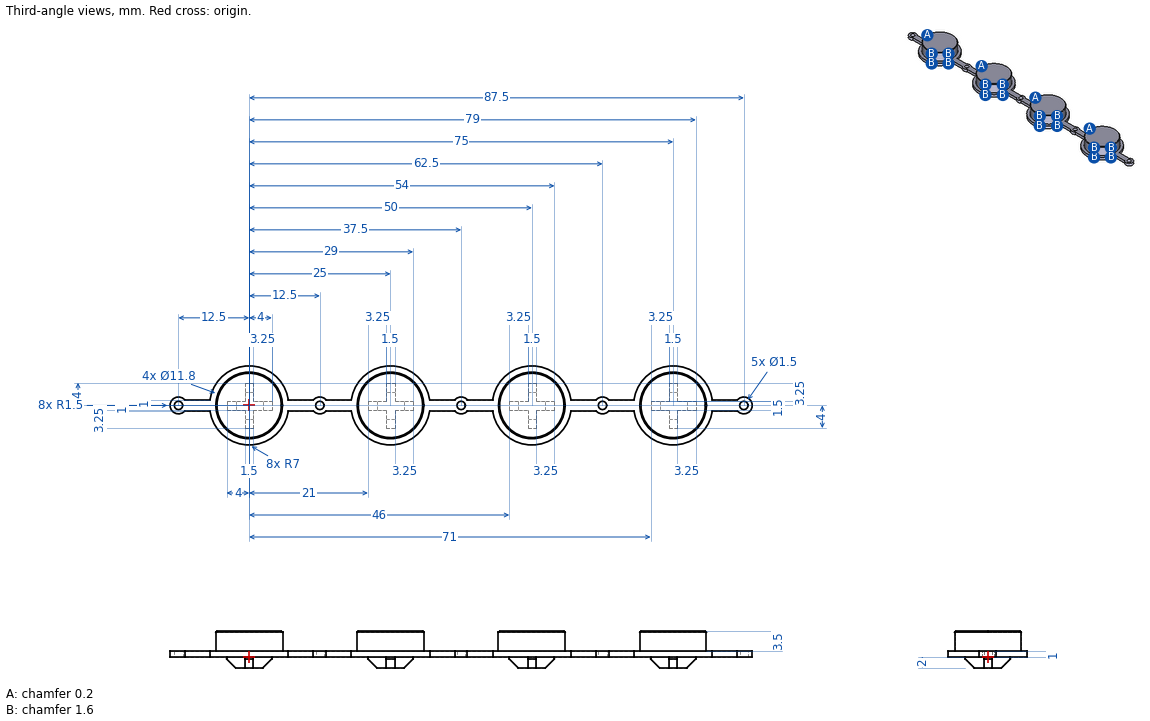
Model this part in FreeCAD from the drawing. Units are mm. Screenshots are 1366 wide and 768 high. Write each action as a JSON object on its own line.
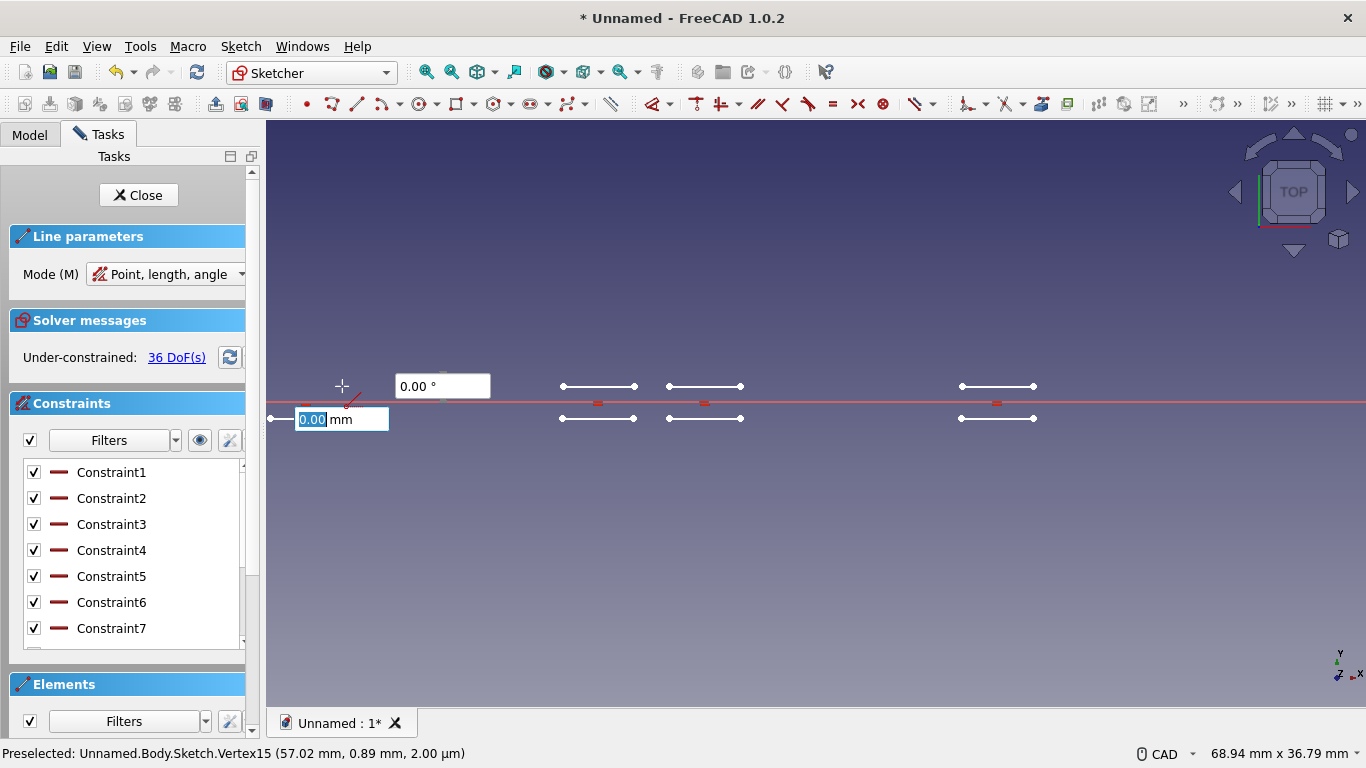
{"action": "scroll", "coordinate": [1036, 420], "scroll_direction": "down", "scroll_amount": 5}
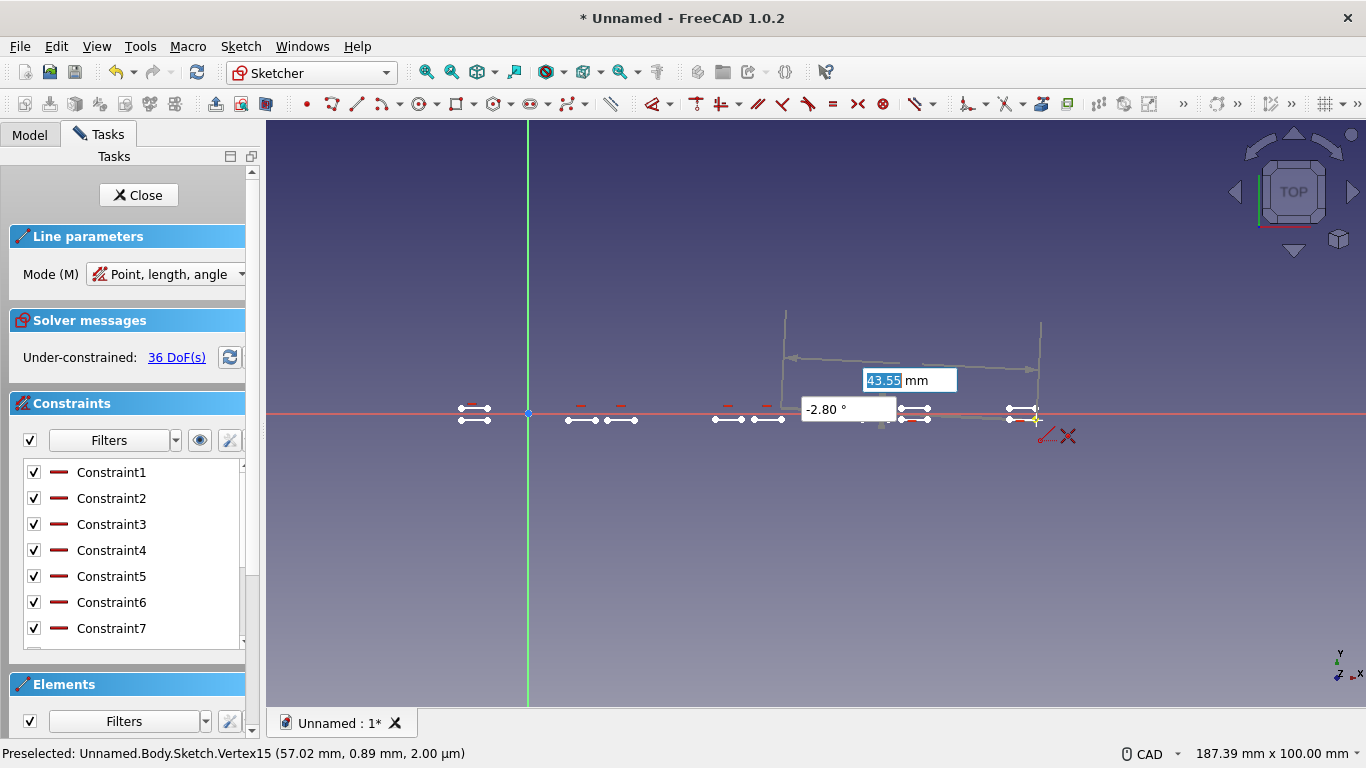
{"action": "scroll", "coordinate": [755, 408], "scroll_direction": "up", "scroll_amount": 5}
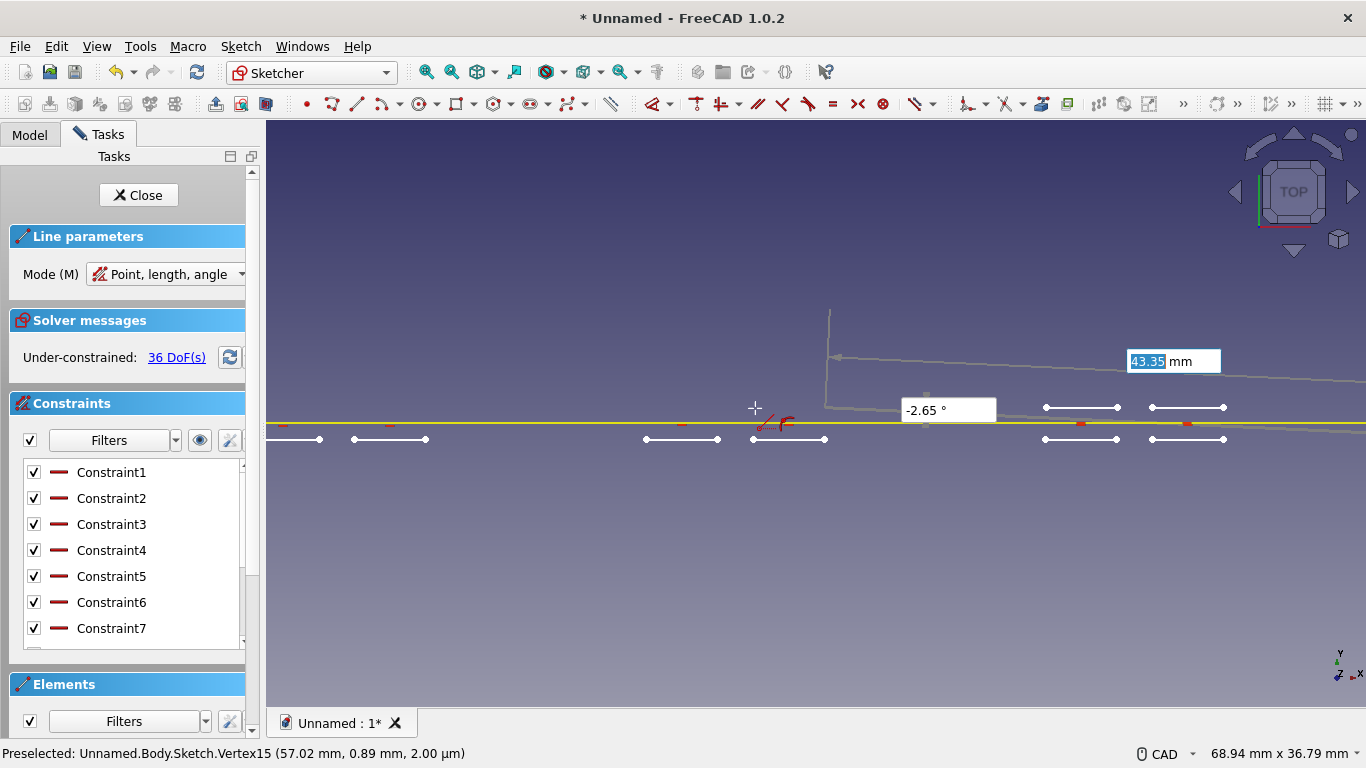
{"action": "left_click", "coordinate": [754, 407]}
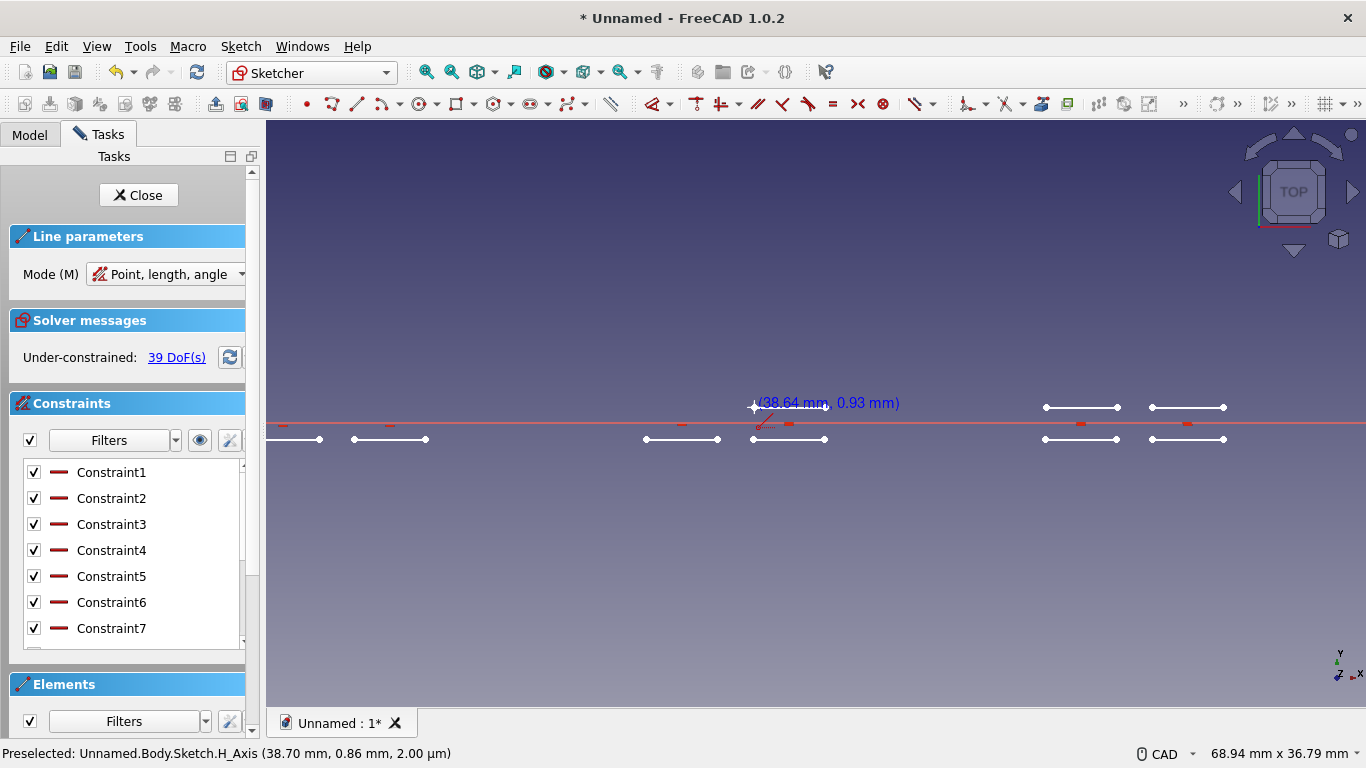
{"action": "left_click", "coordinate": [718, 407]}
{"action": "left_click", "coordinate": [647, 407]}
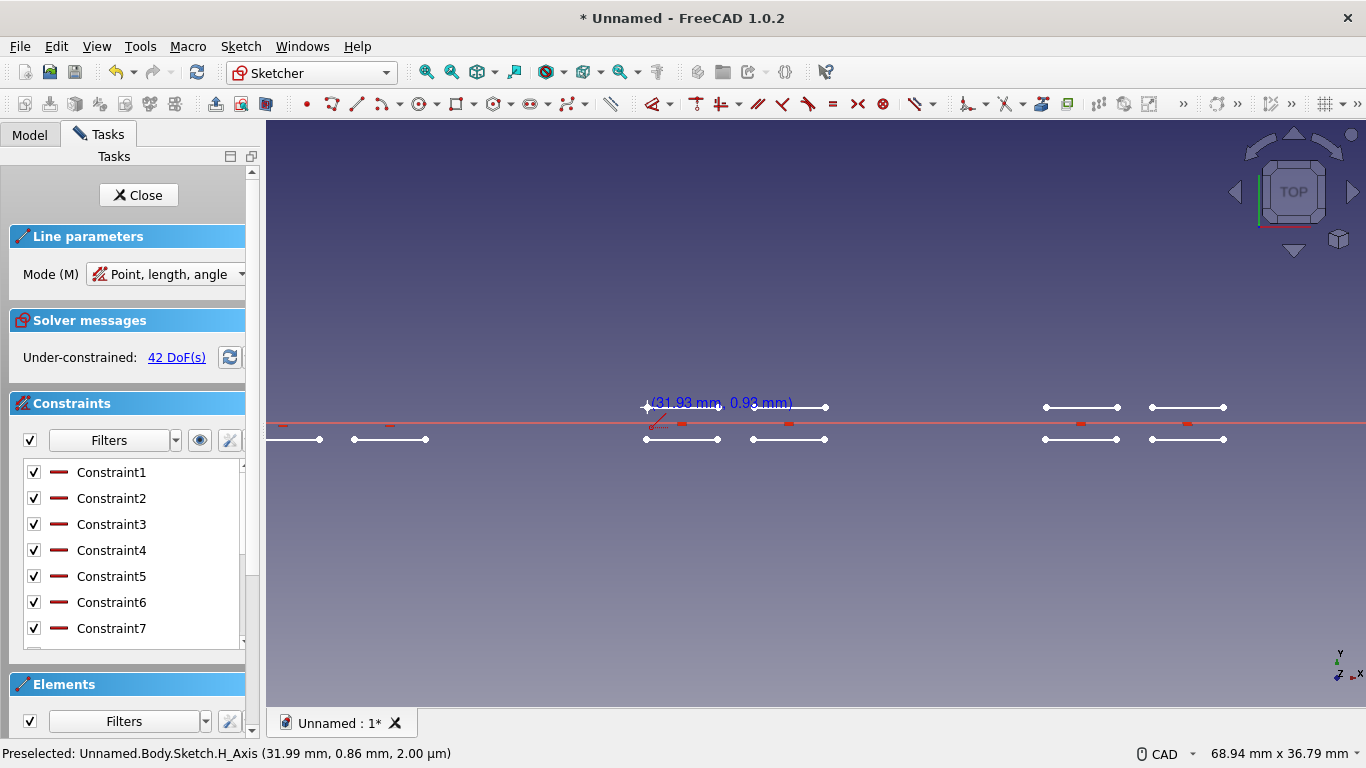
{"action": "left_click", "coordinate": [426, 407]}
{"action": "left_click", "coordinate": [355, 407]}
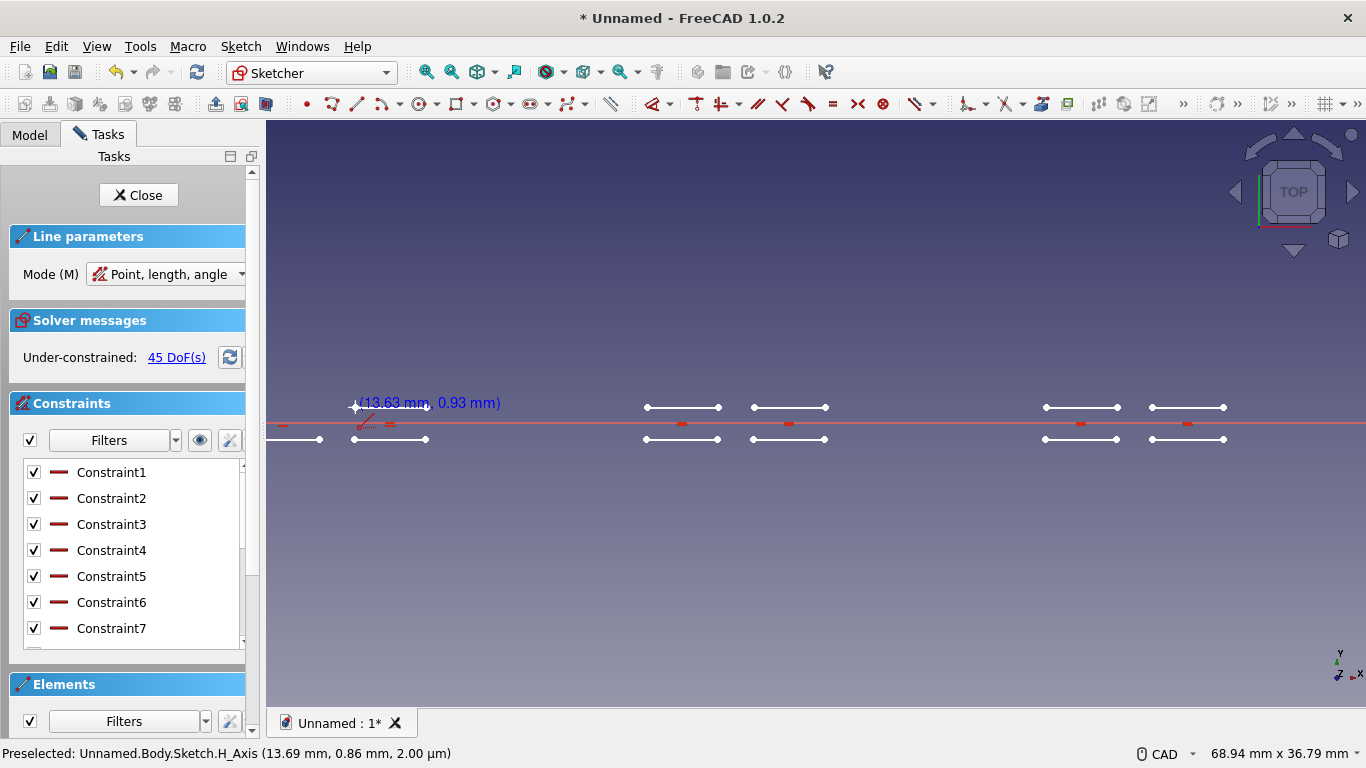
{"action": "left_click", "coordinate": [319, 407]}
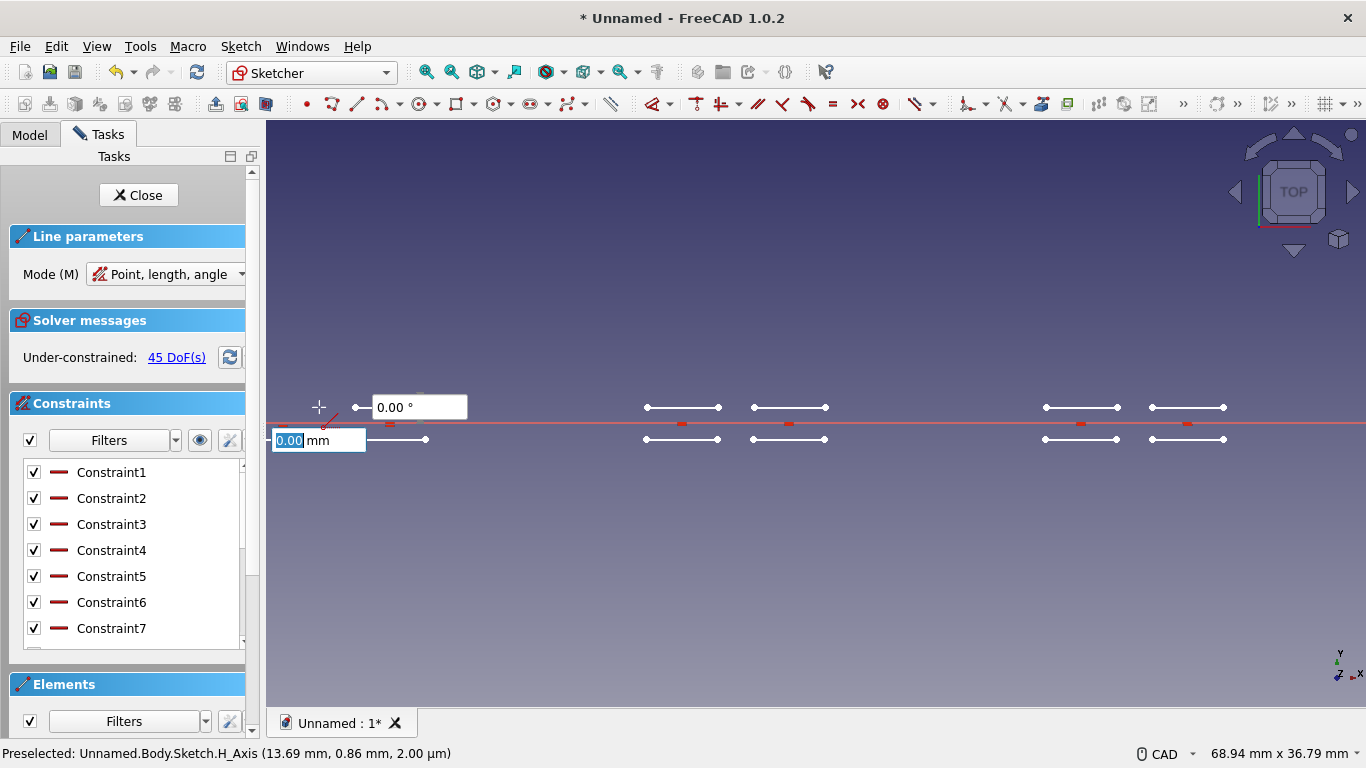
{"action": "scroll", "coordinate": [754, 408], "scroll_direction": "down", "scroll_amount": 5}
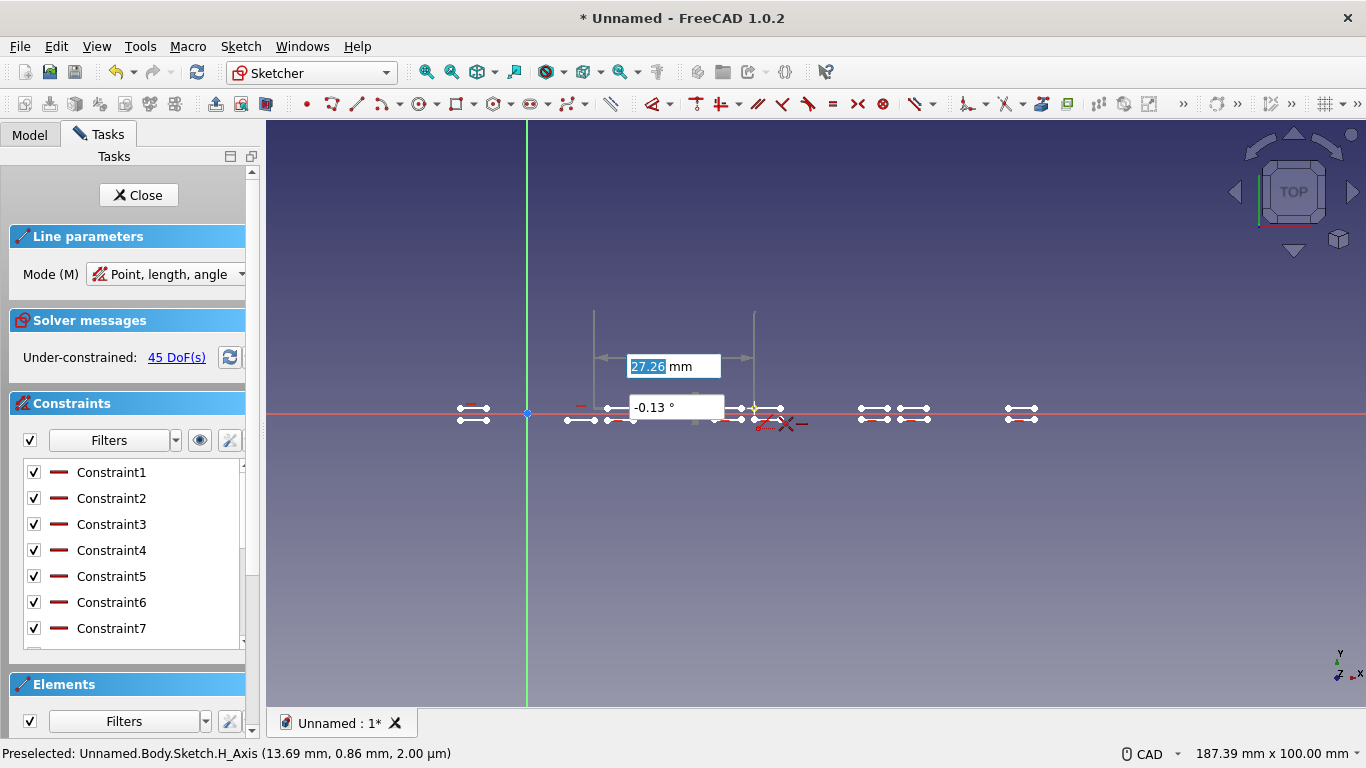
{"action": "scroll", "coordinate": [568, 408], "scroll_direction": "up", "scroll_amount": 5}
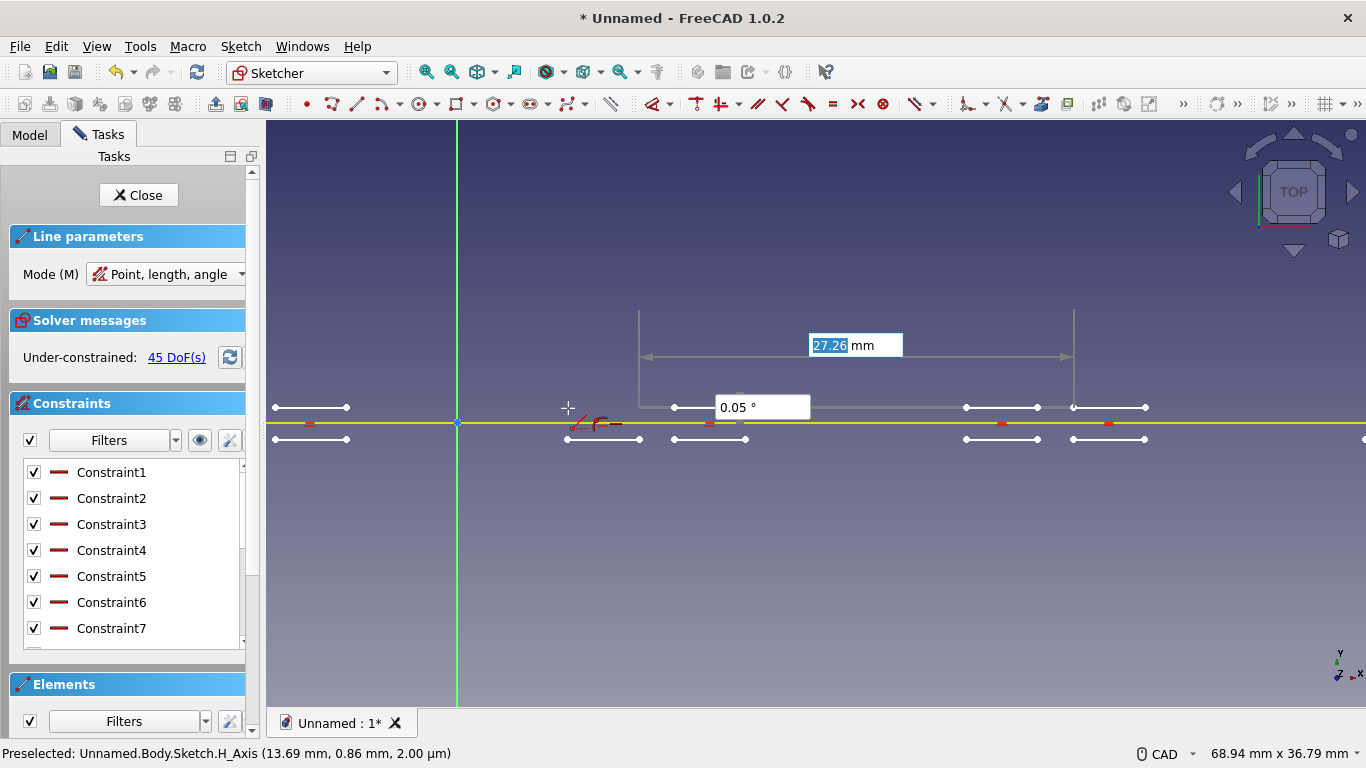
{"action": "left_click", "coordinate": [568, 407]}